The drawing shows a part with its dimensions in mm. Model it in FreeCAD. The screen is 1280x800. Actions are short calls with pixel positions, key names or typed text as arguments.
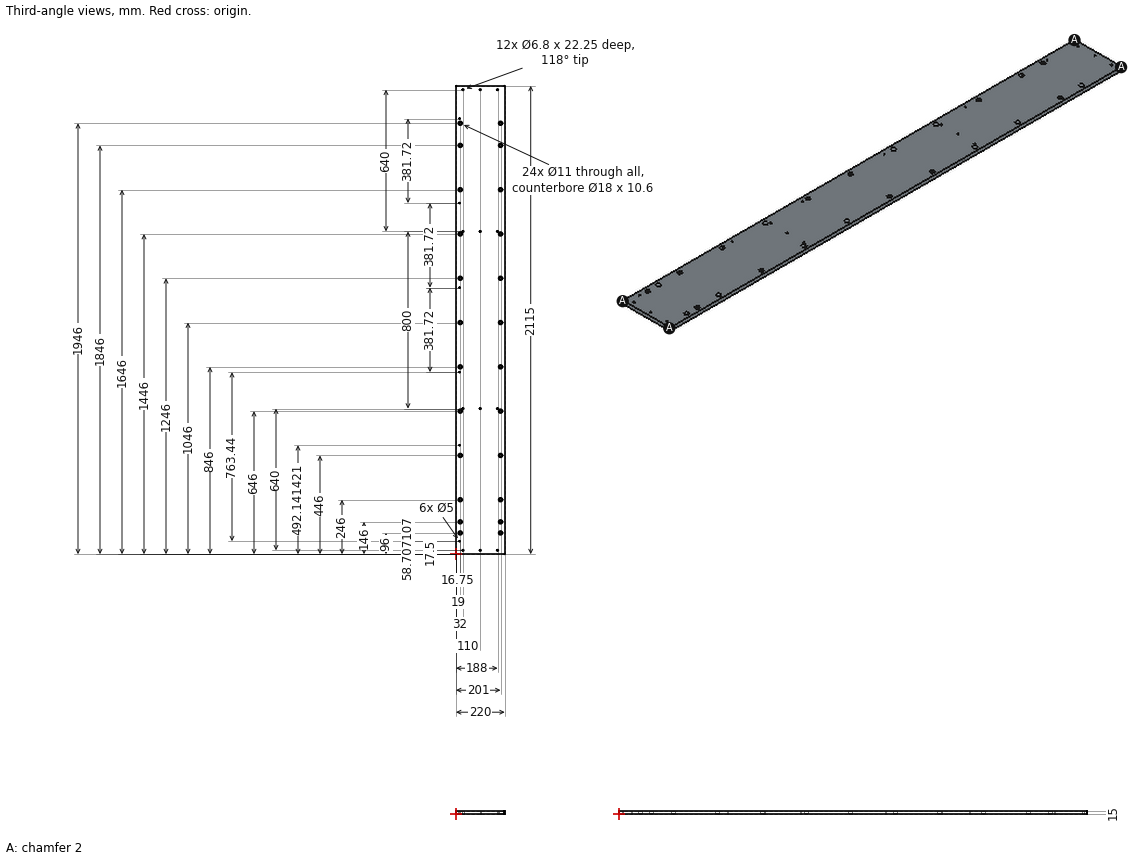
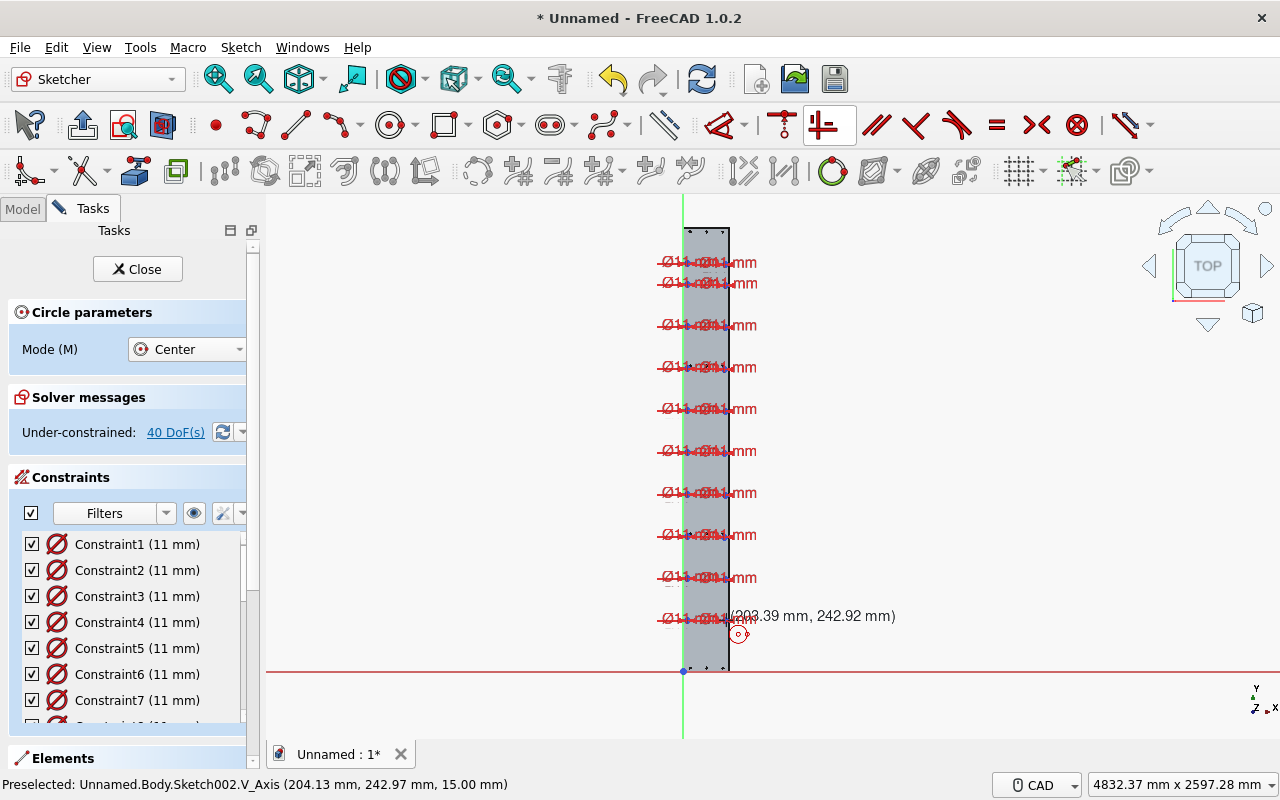
scroll(687, 641, up, 15)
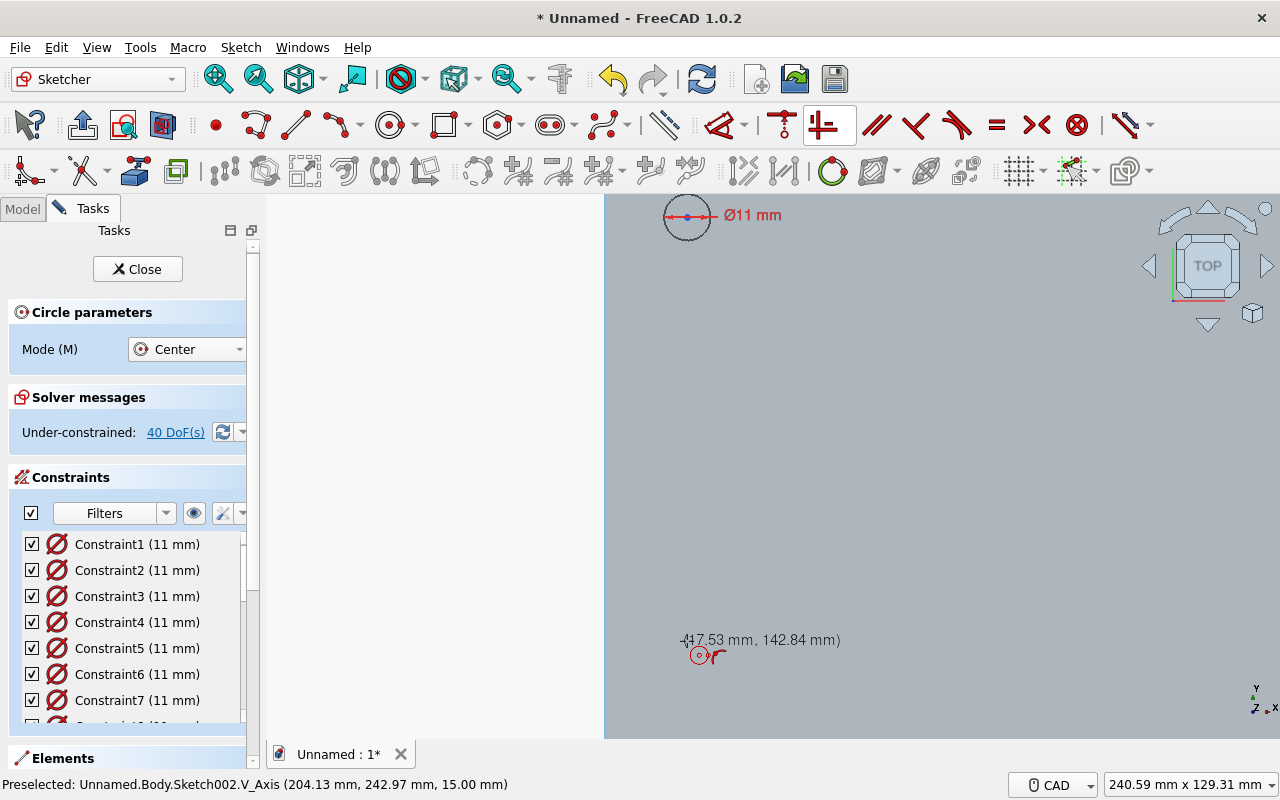
scroll(687, 641, down, 15)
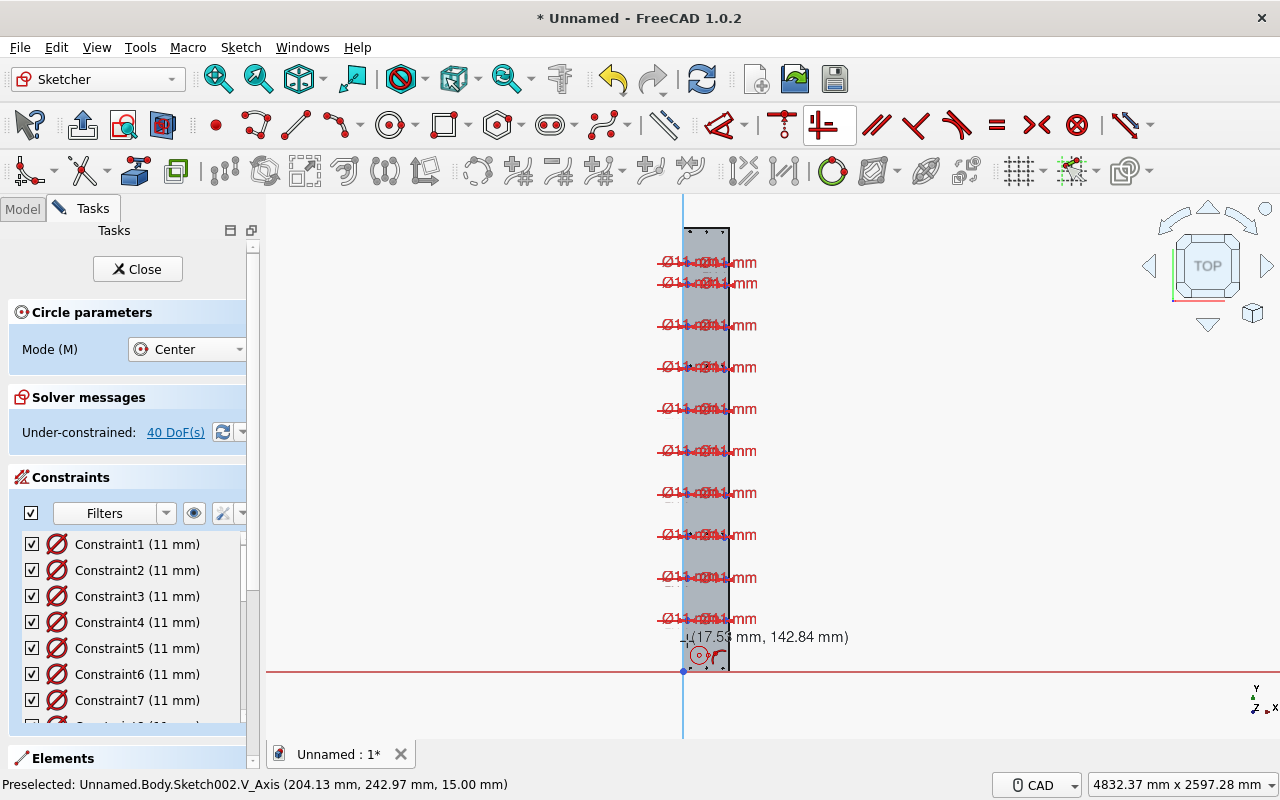
scroll(687, 641, up, 7)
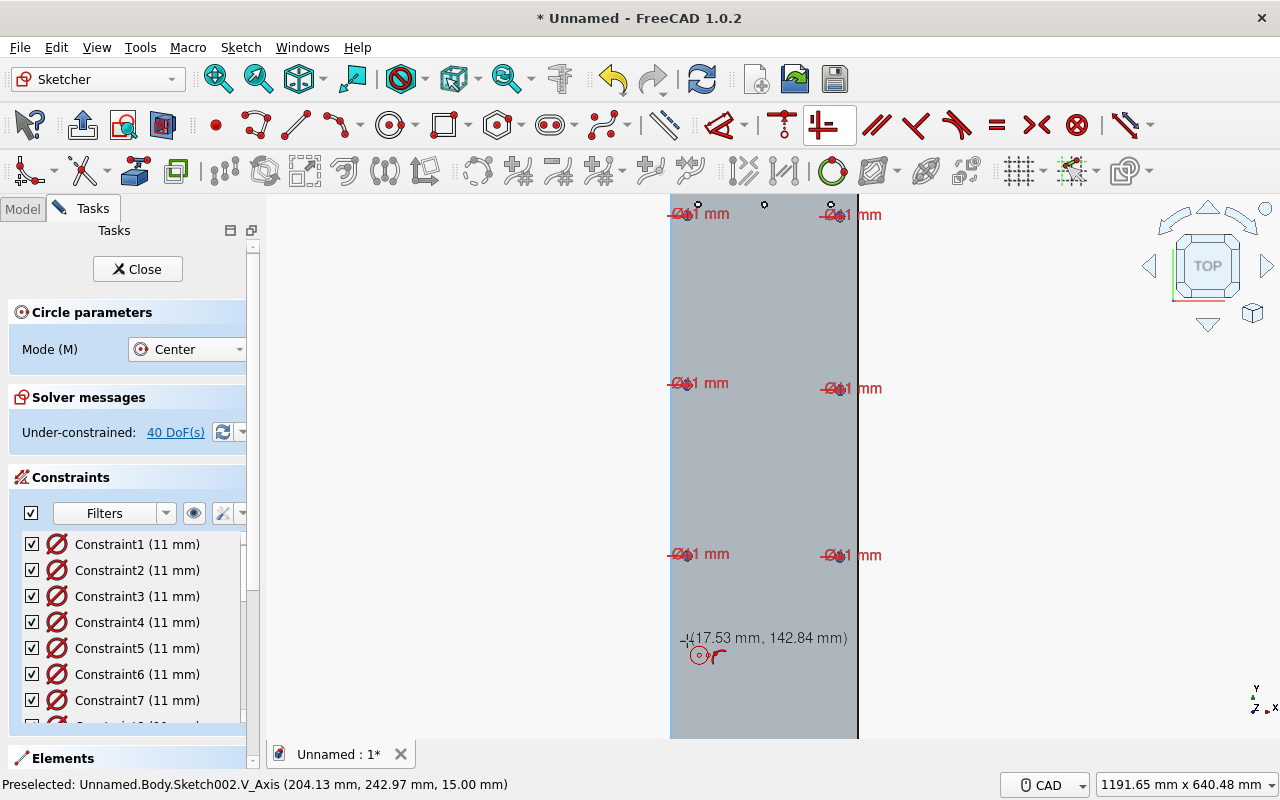
click(687, 640)
move(690, 637)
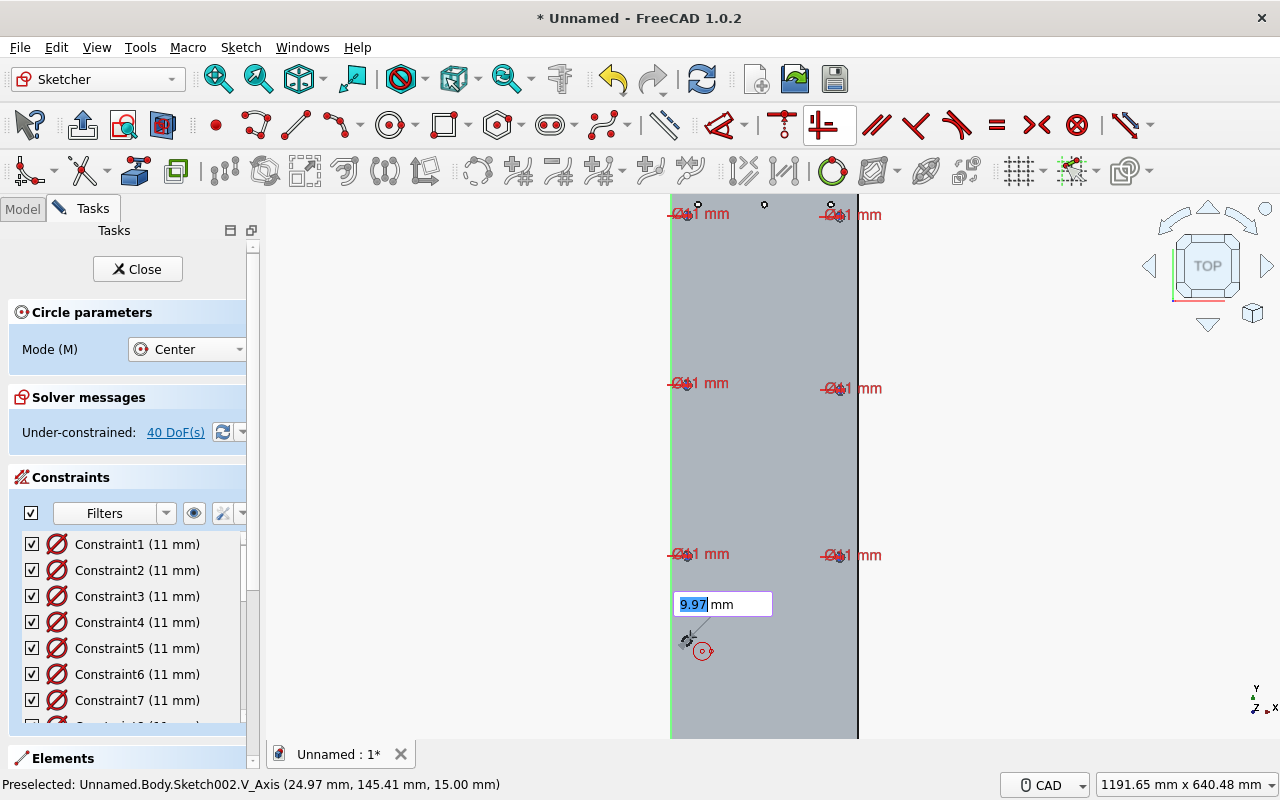
text(11)
key(Return)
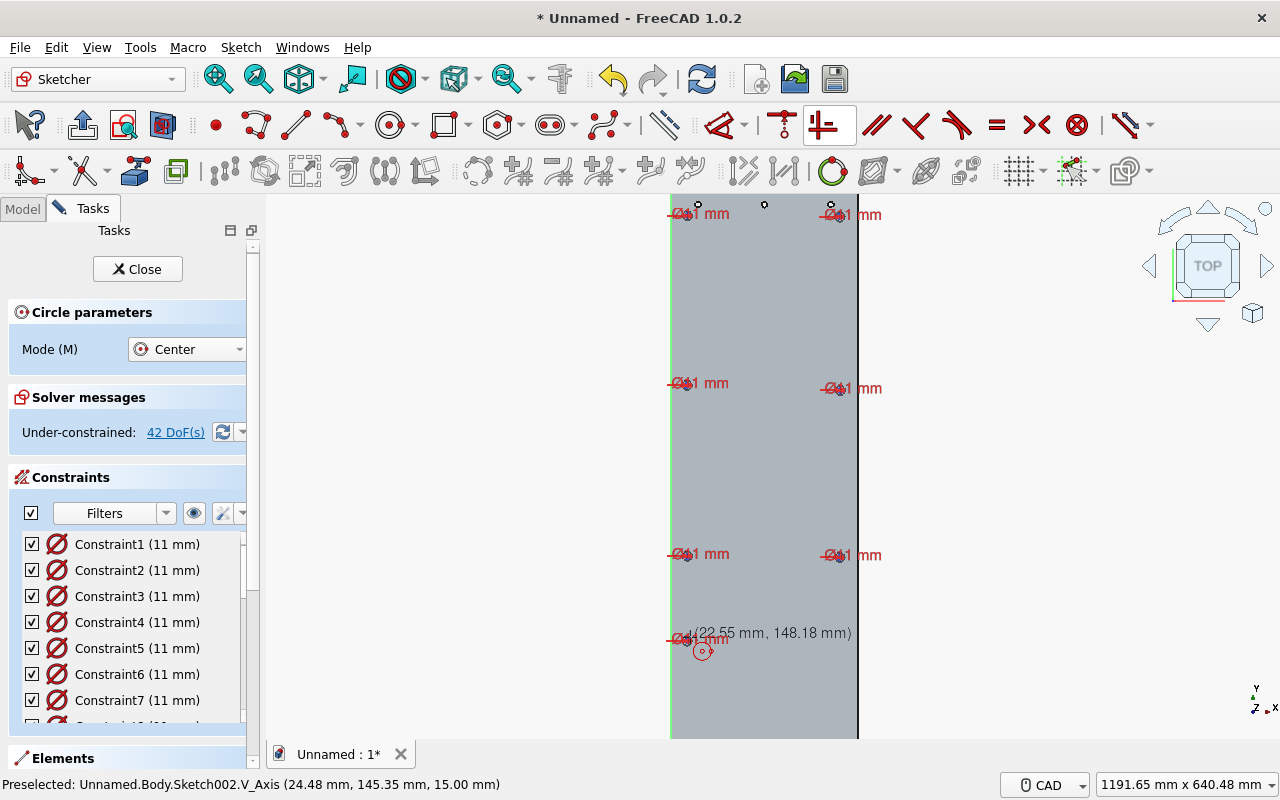
scroll(842, 640, up, 8)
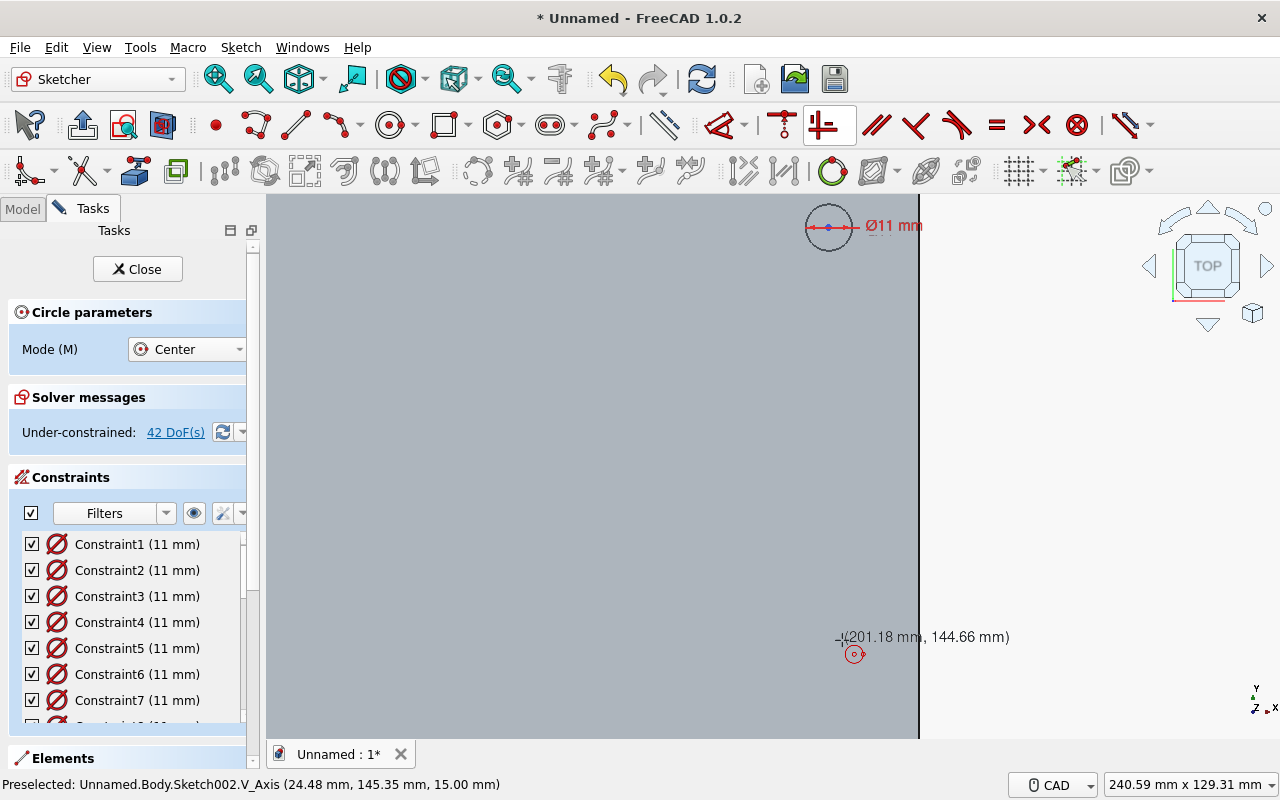
scroll(719, 641, down, 15)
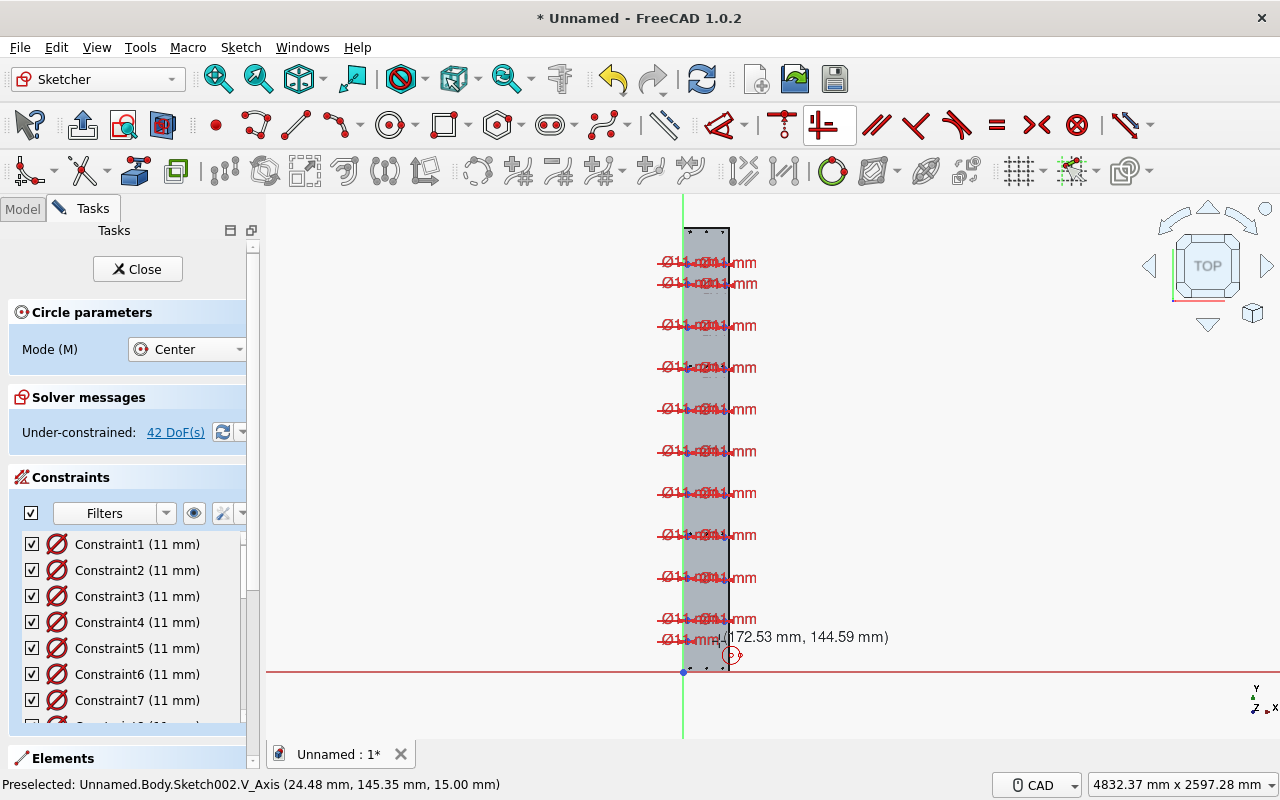
click(725, 642)
move(726, 641)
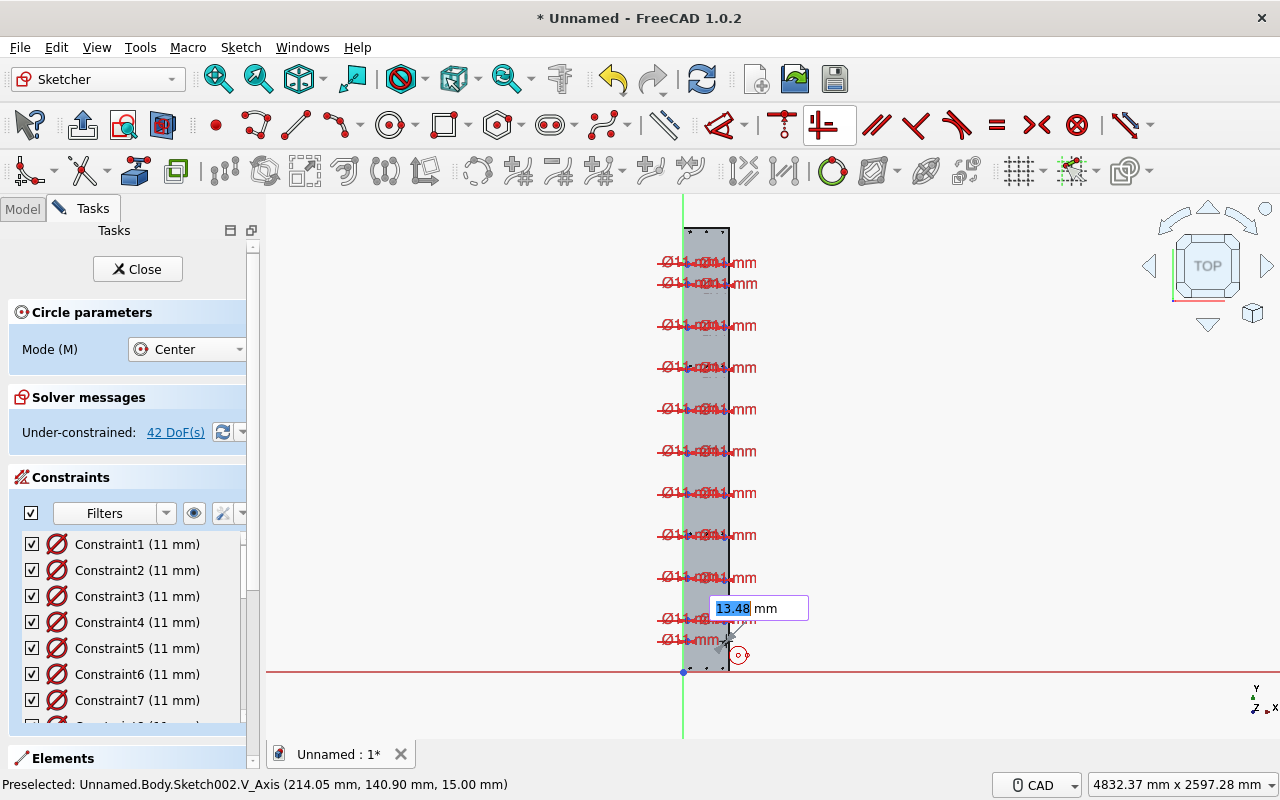
text(11)
key(Return)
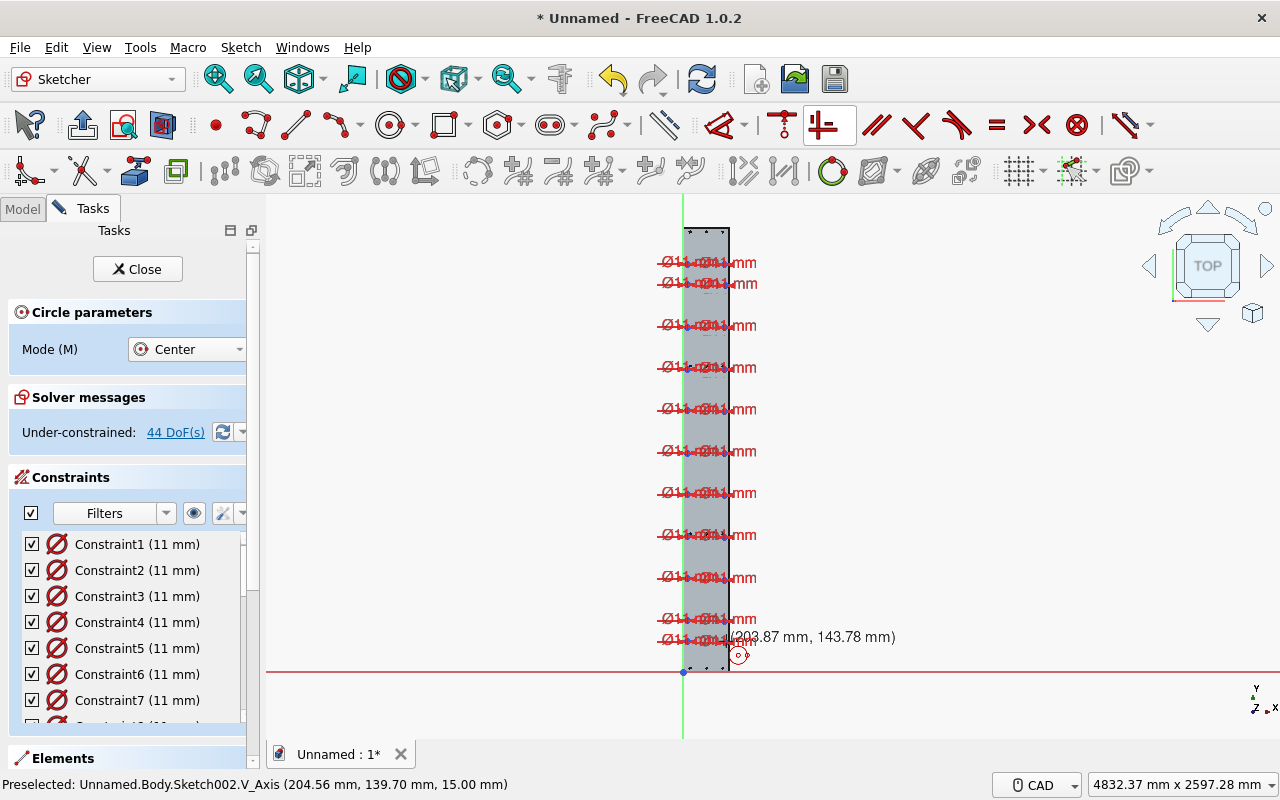
scroll(687, 652, up, 15)